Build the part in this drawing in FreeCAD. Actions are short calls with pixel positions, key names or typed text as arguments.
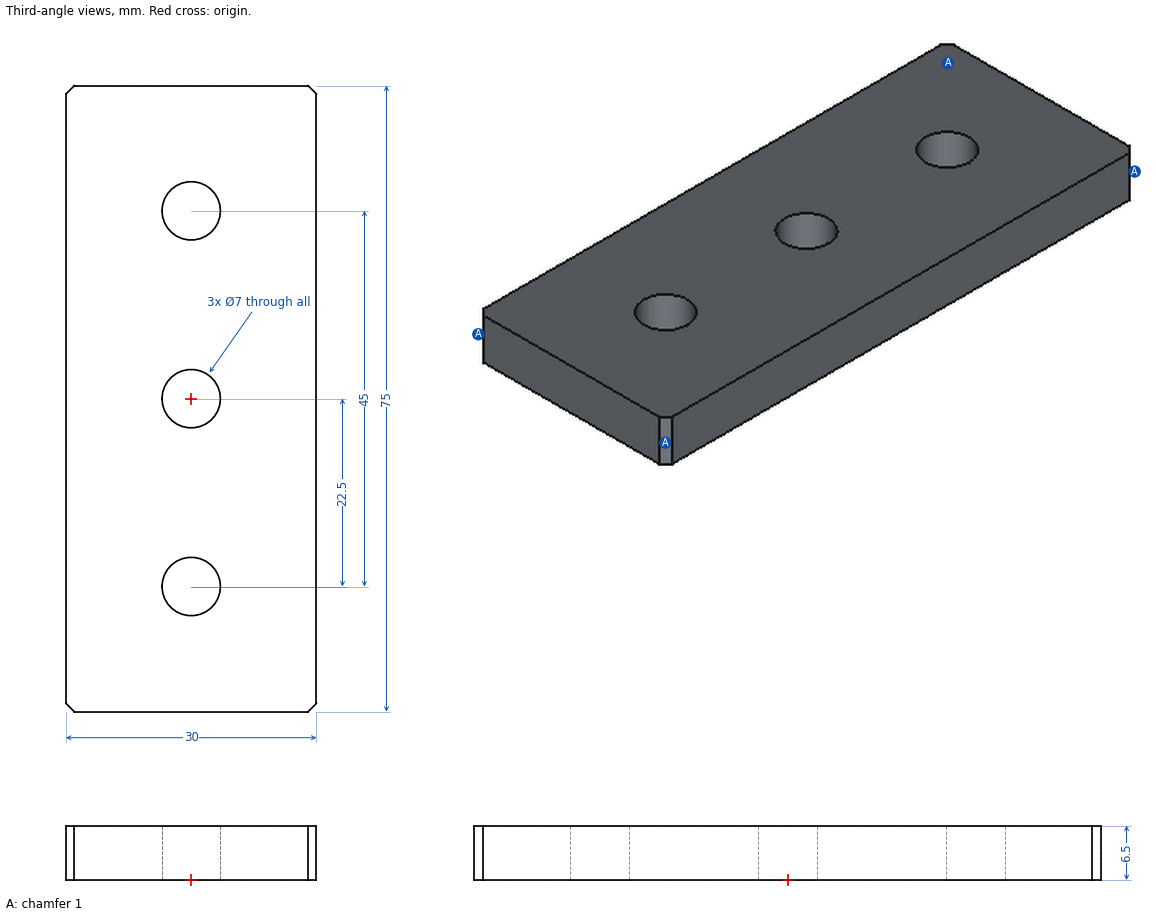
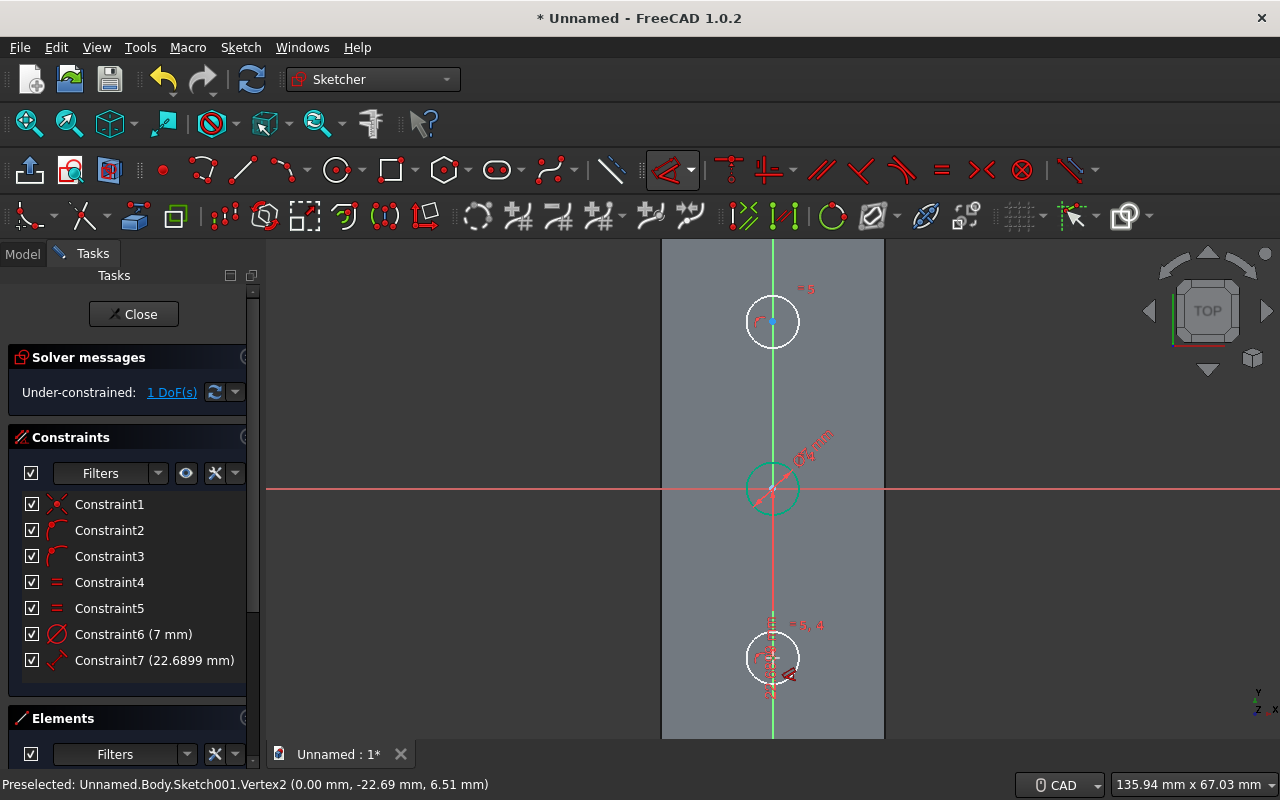
click(773, 322)
click(807, 413)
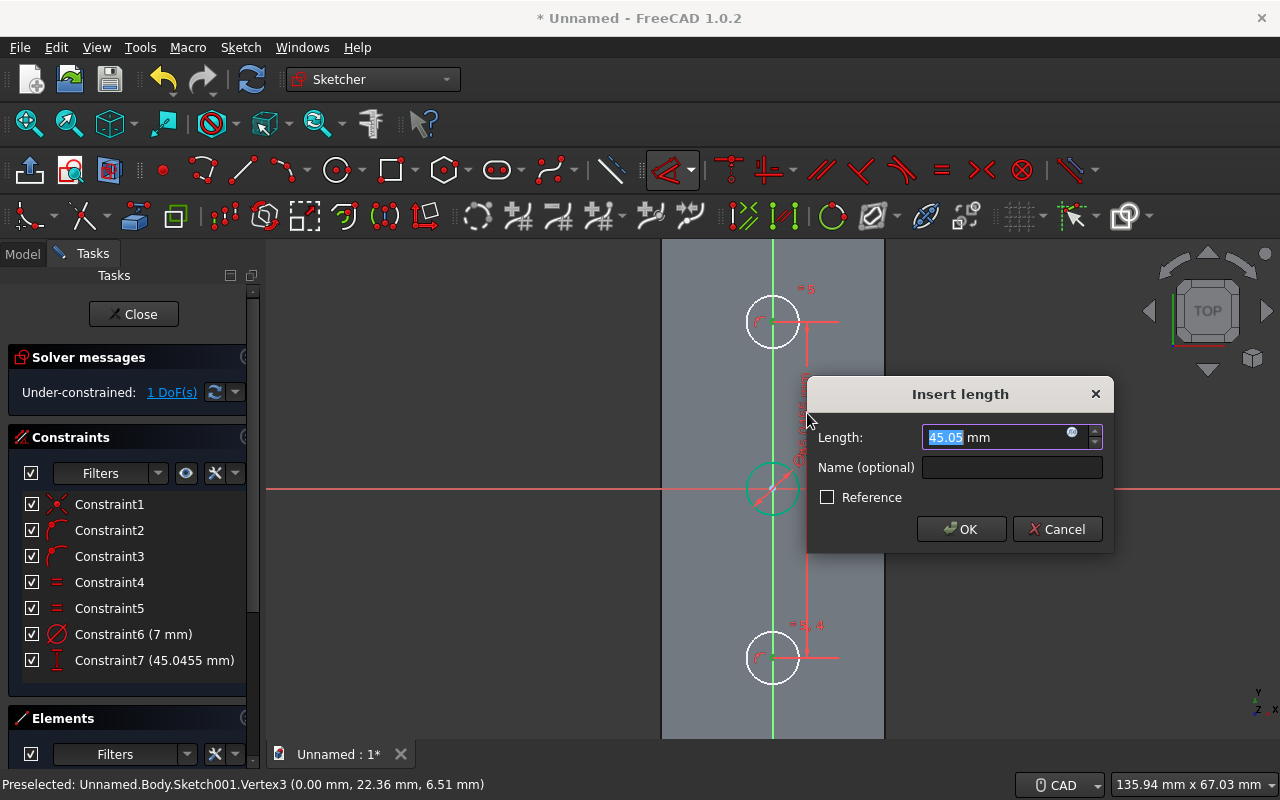
text(45)
key(Return)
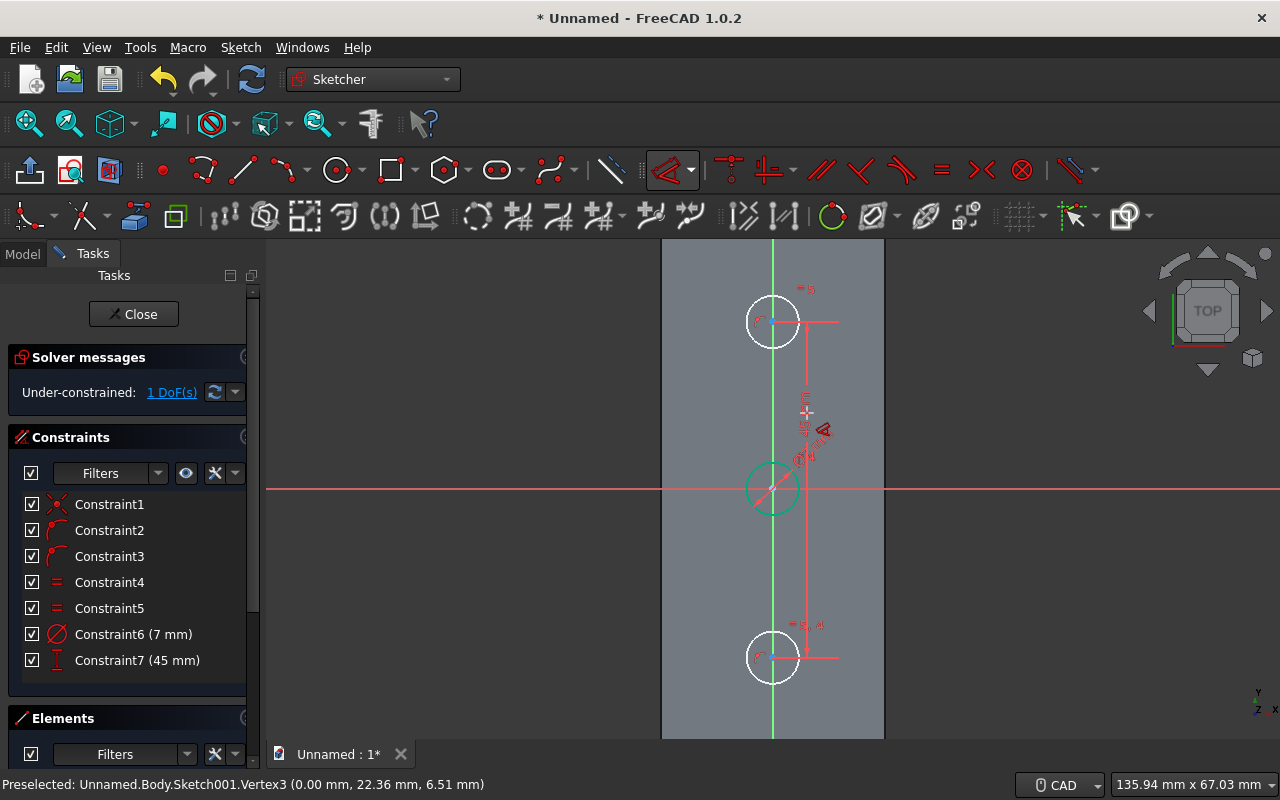
click(773, 658)
click(807, 573)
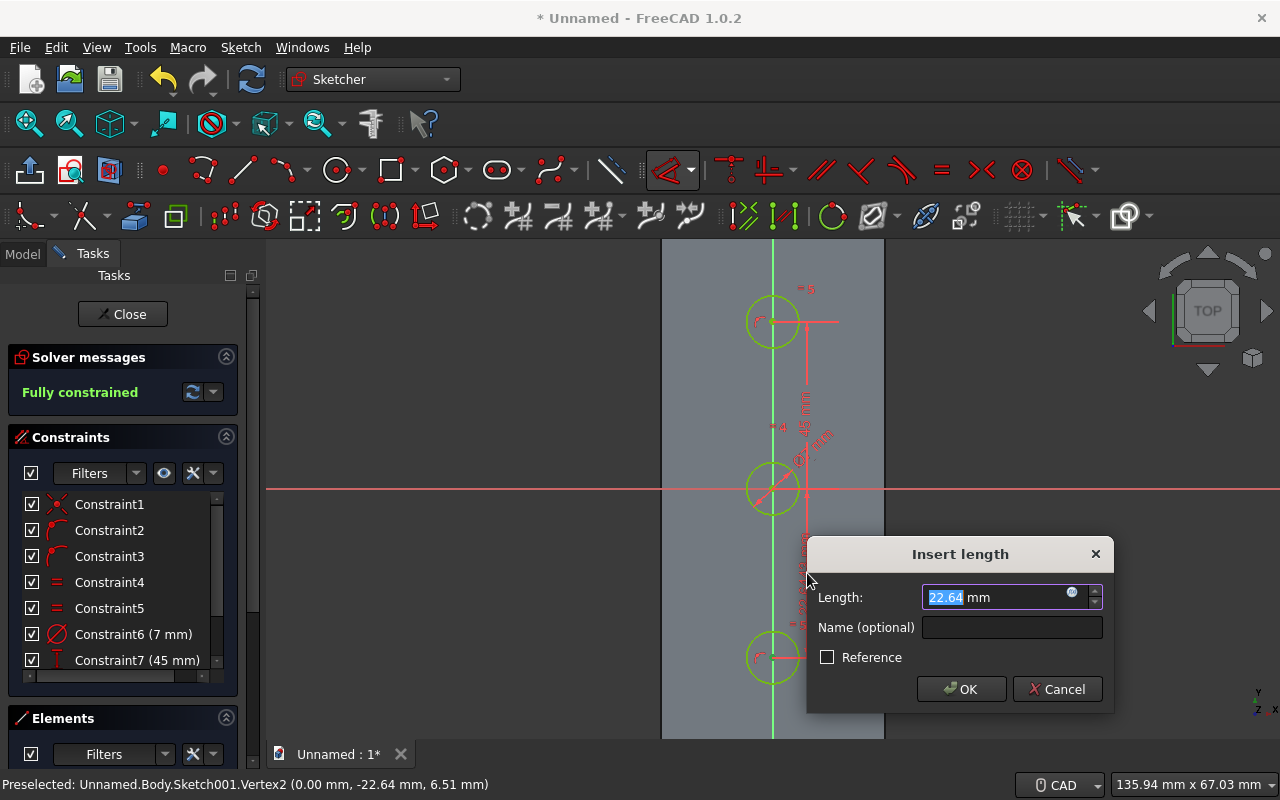
text(22.5)
key(Return)
key(Escape)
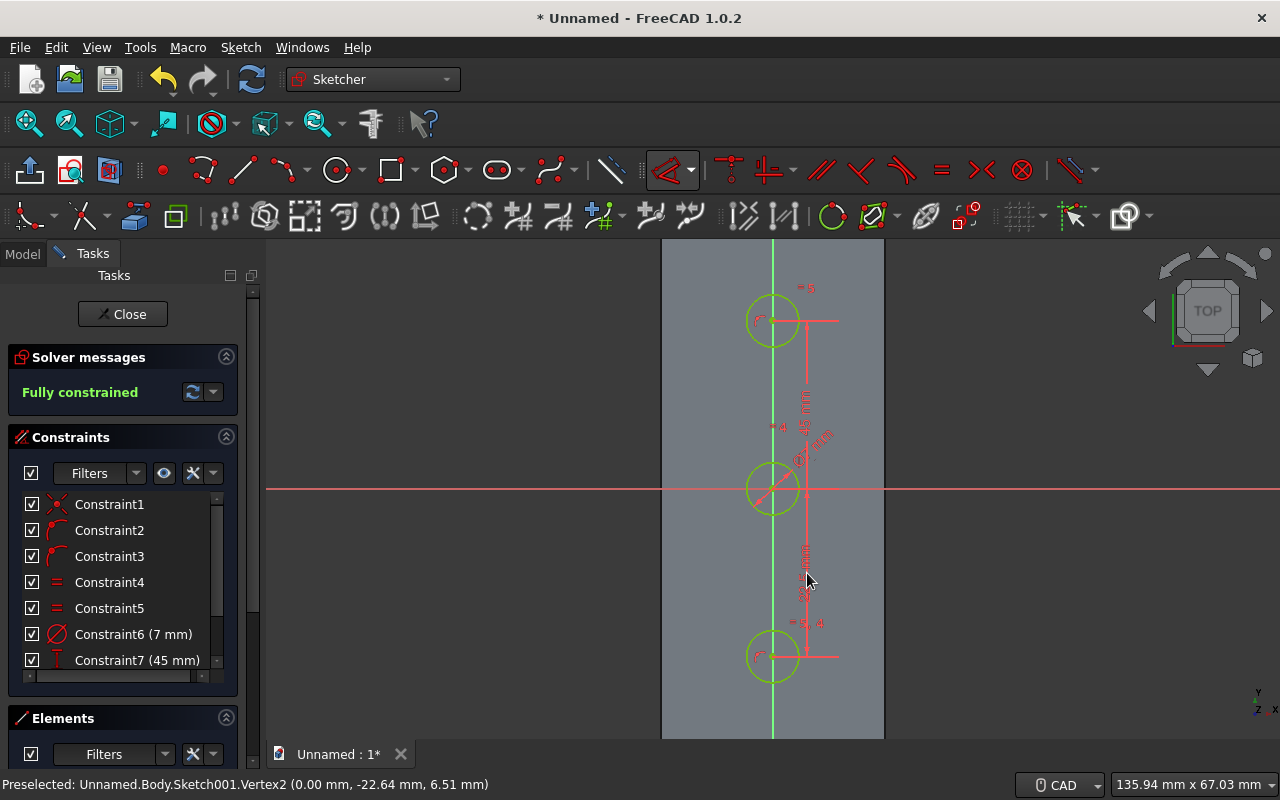
click(123, 314)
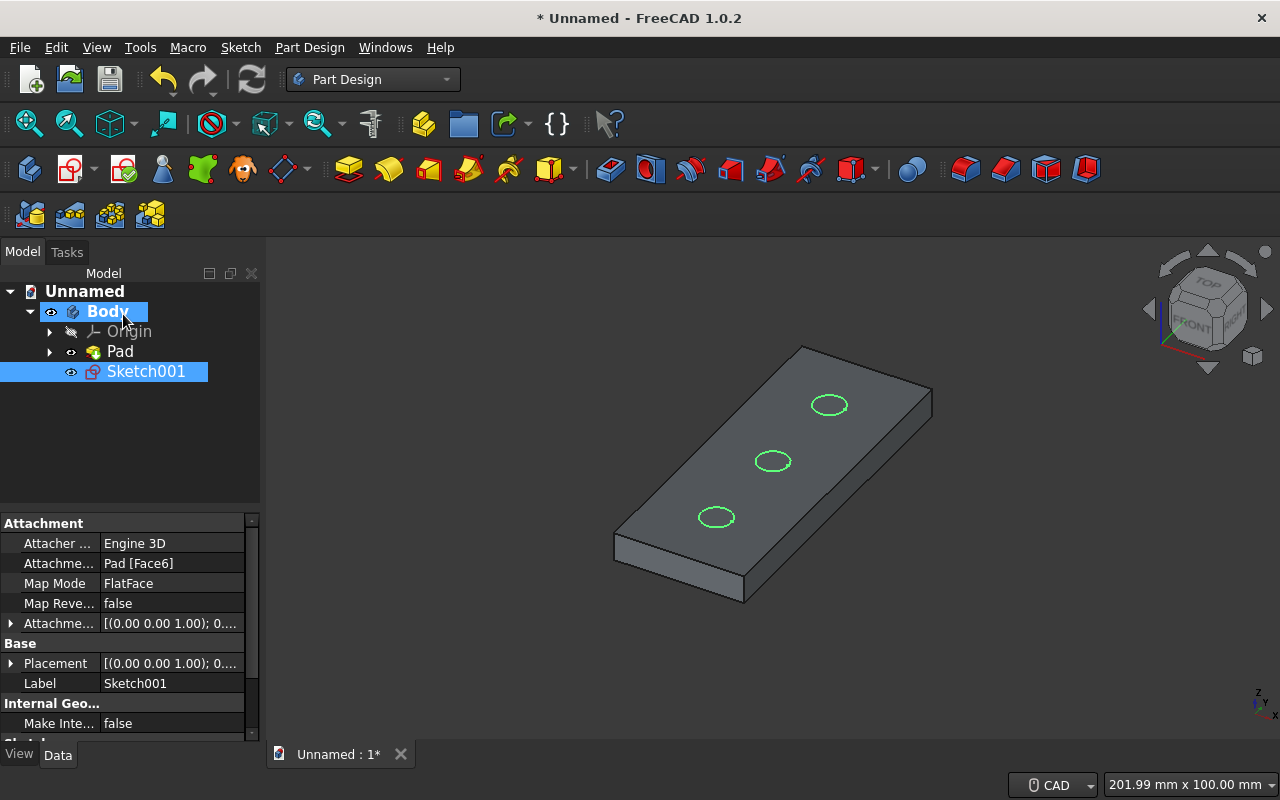
click(652, 170)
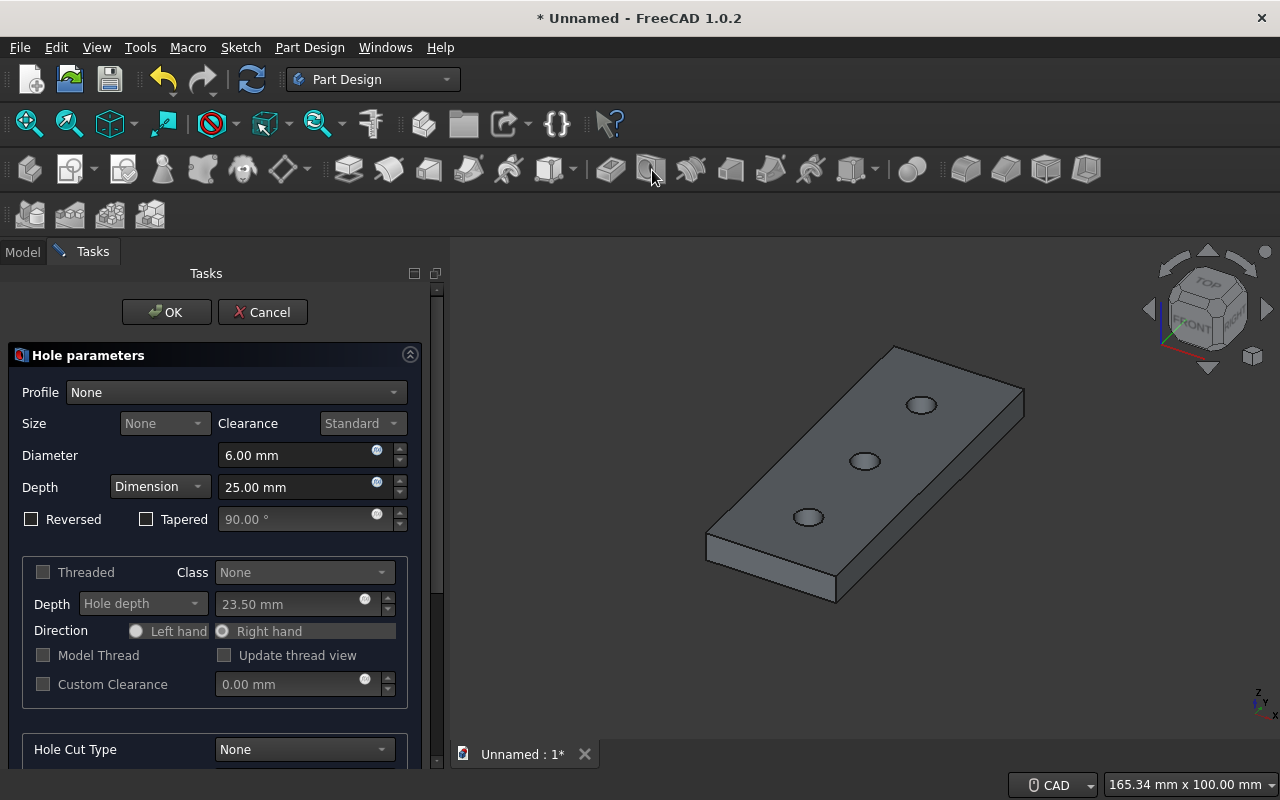
triple_click(305, 455)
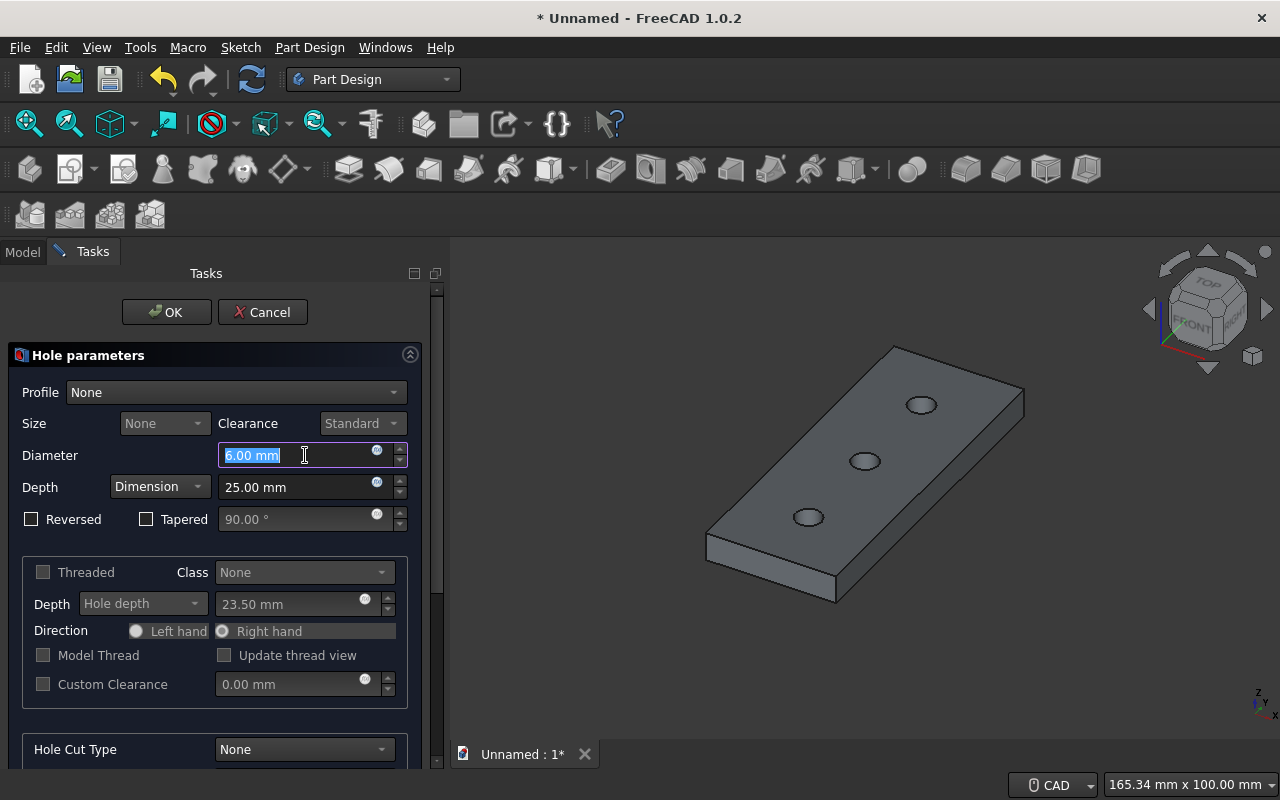
text(7)
key(Tab)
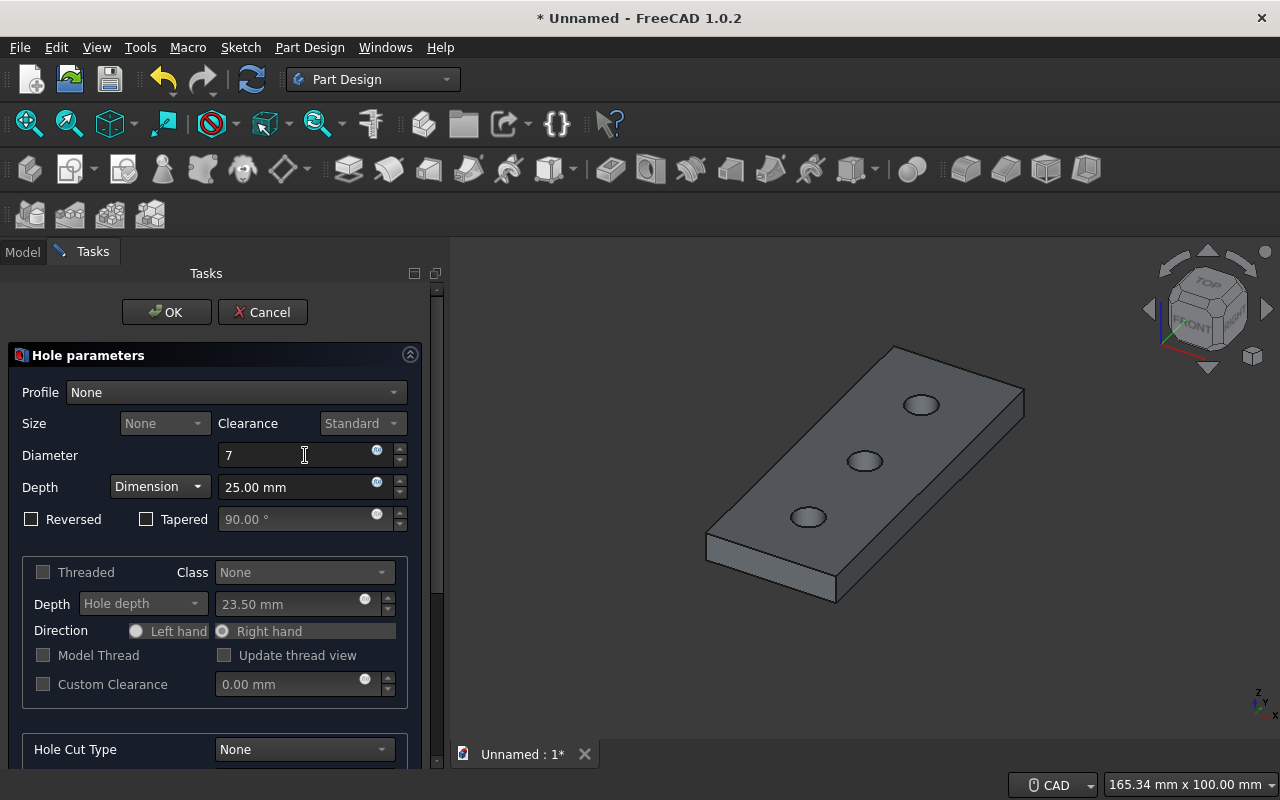
click(161, 486)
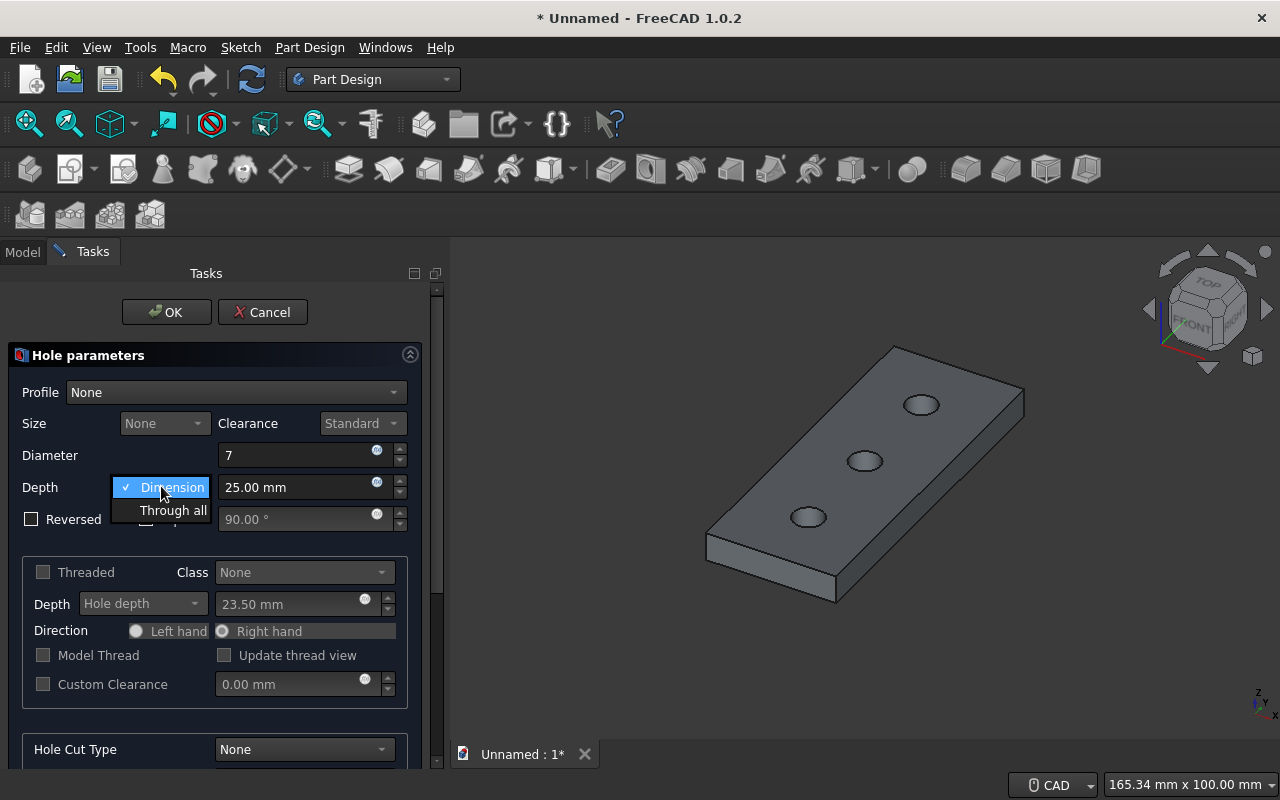
click(160, 510)